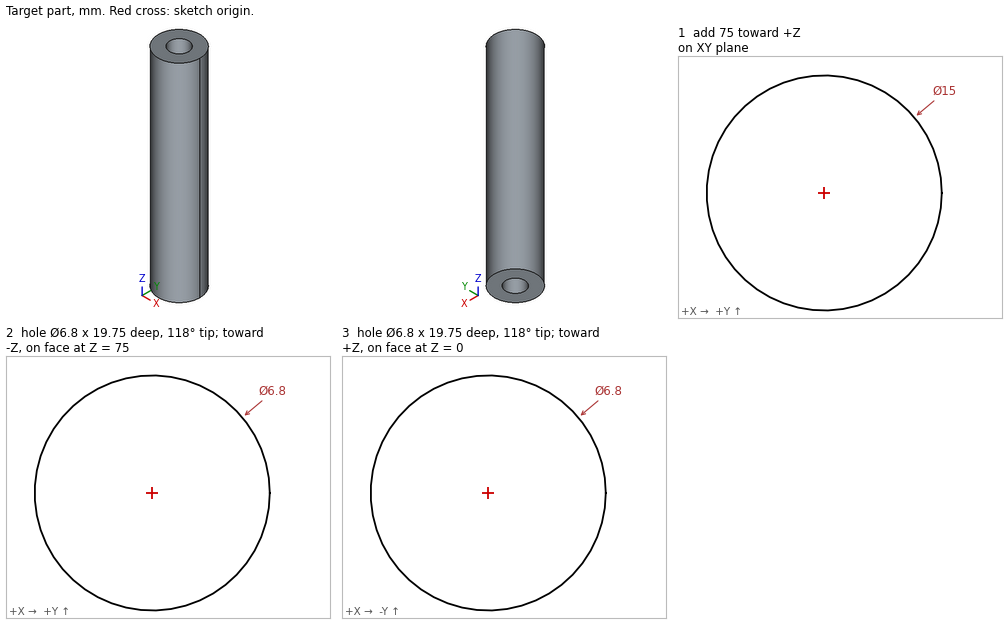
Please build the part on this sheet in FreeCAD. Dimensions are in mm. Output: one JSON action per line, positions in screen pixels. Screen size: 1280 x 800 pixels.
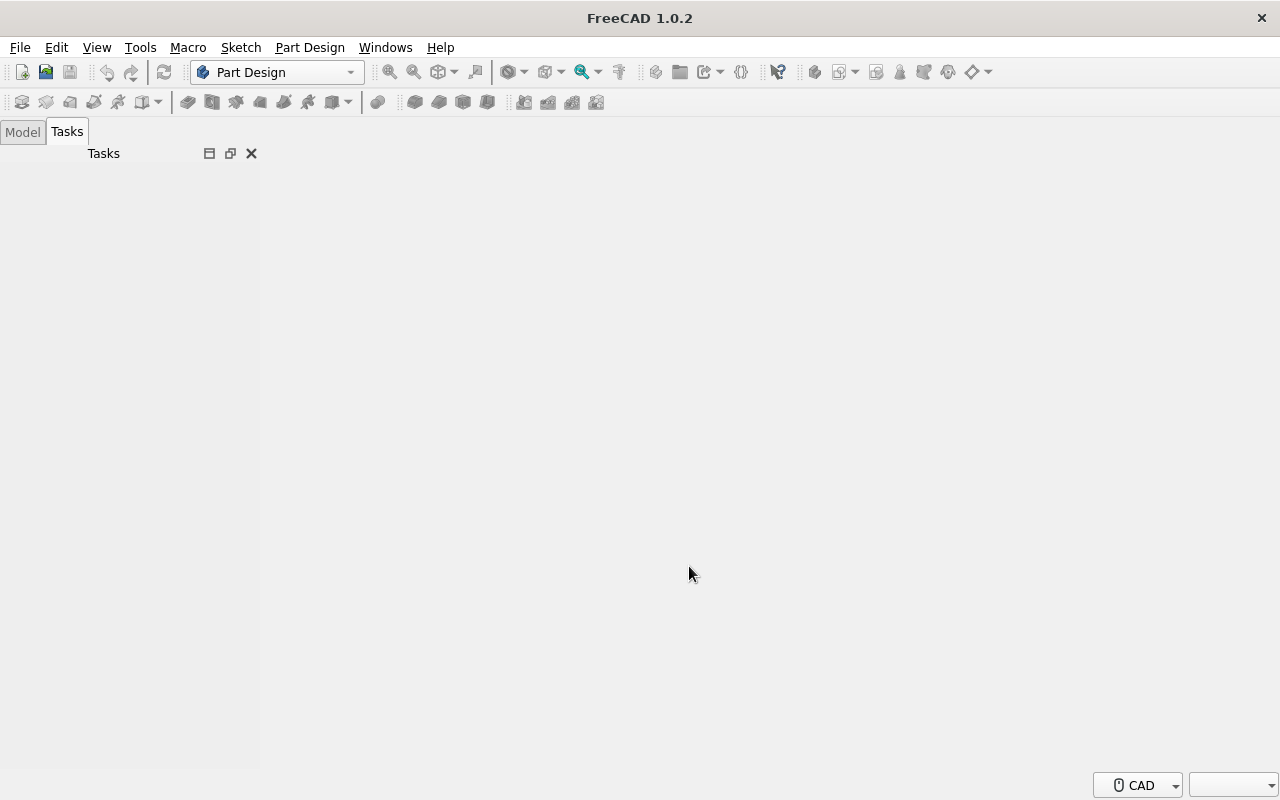
{"action": "left_click", "coordinate": [22, 72]}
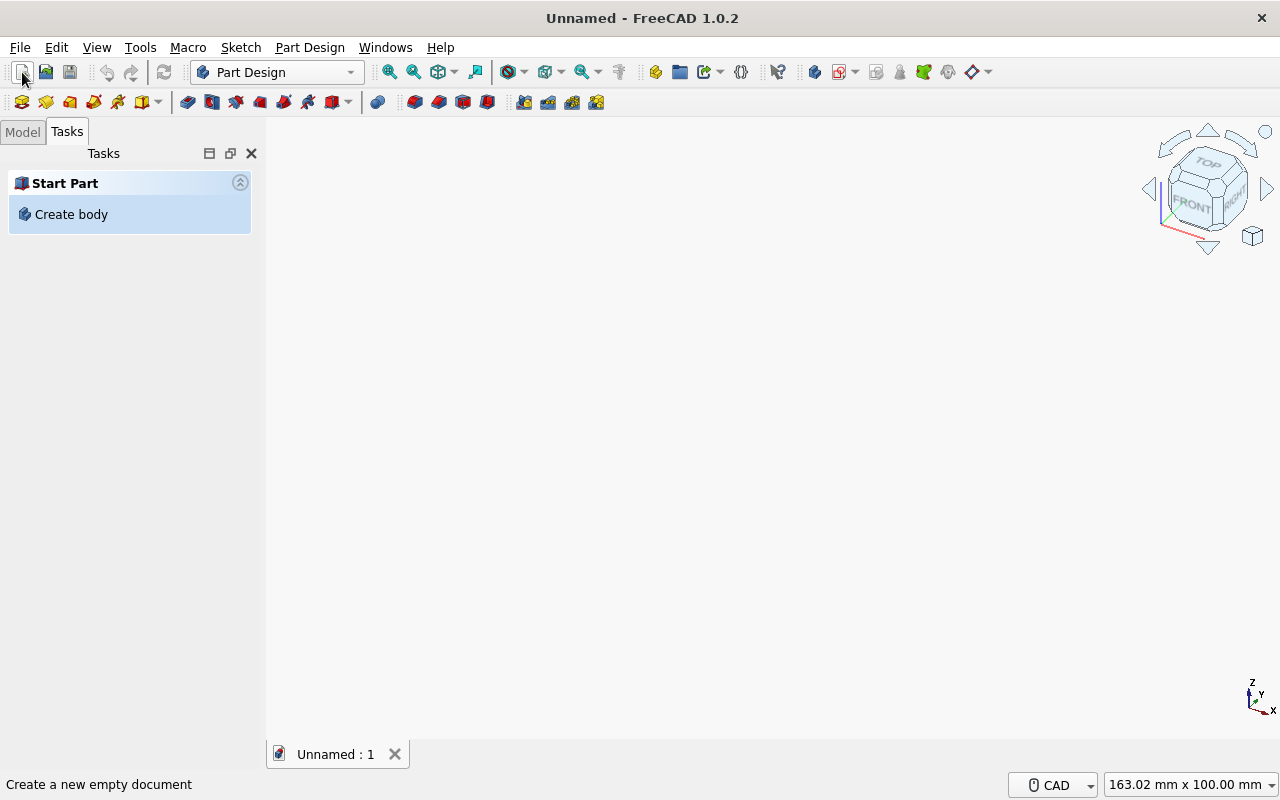
{"action": "left_click", "coordinate": [840, 72]}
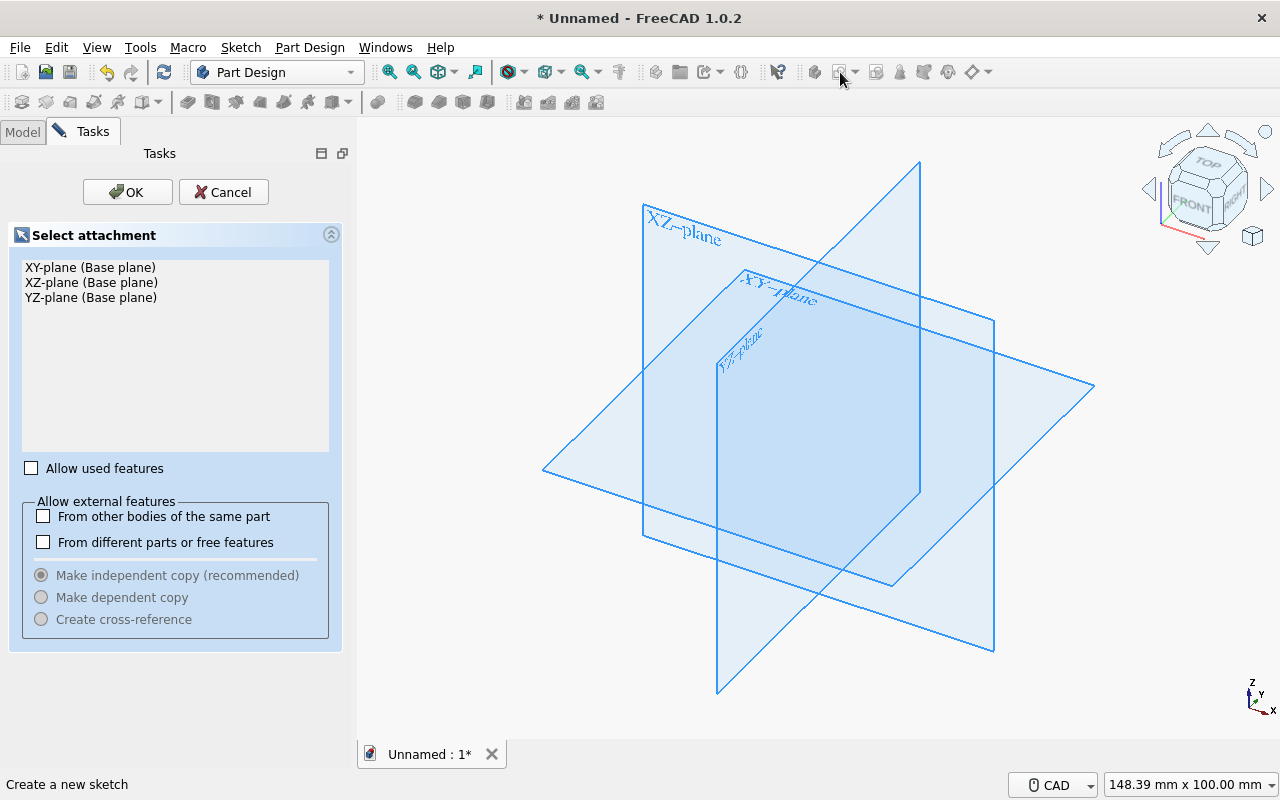
{"action": "left_click", "coordinate": [82, 268]}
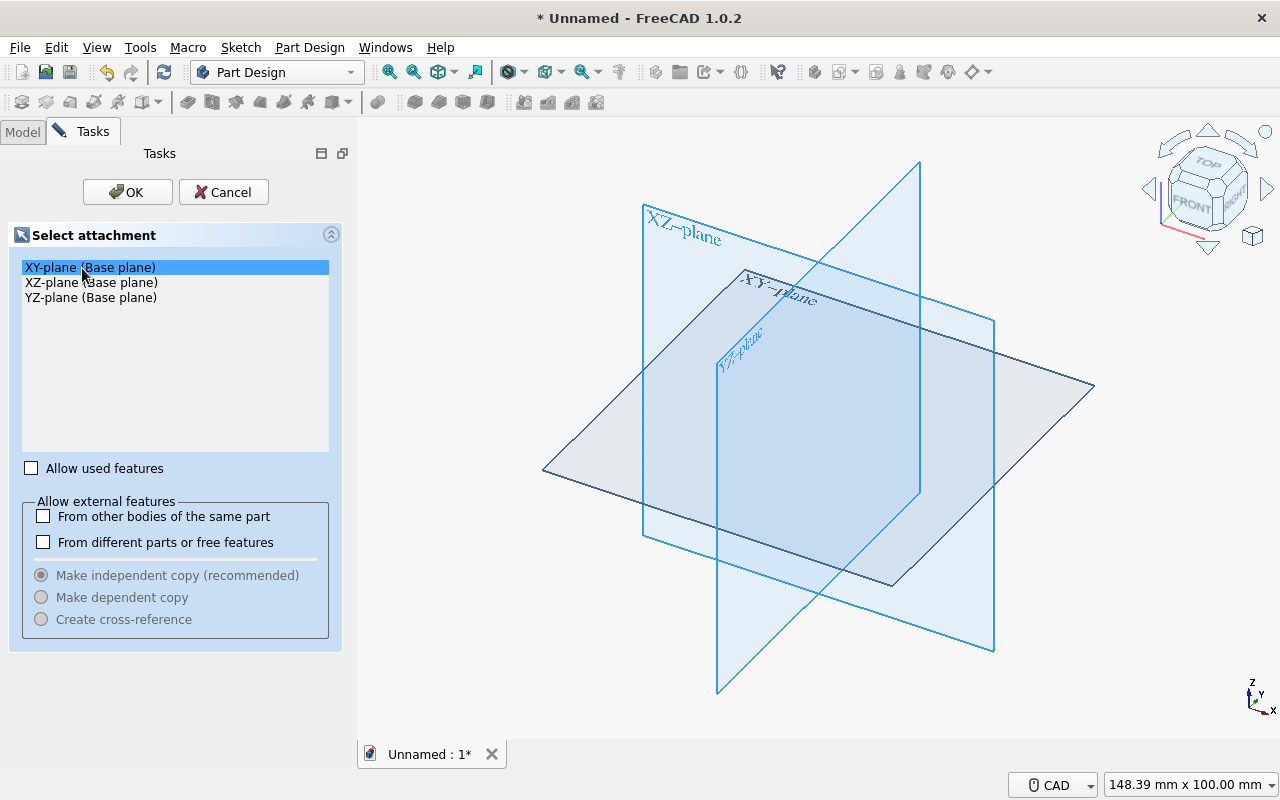
{"action": "left_click", "coordinate": [128, 192]}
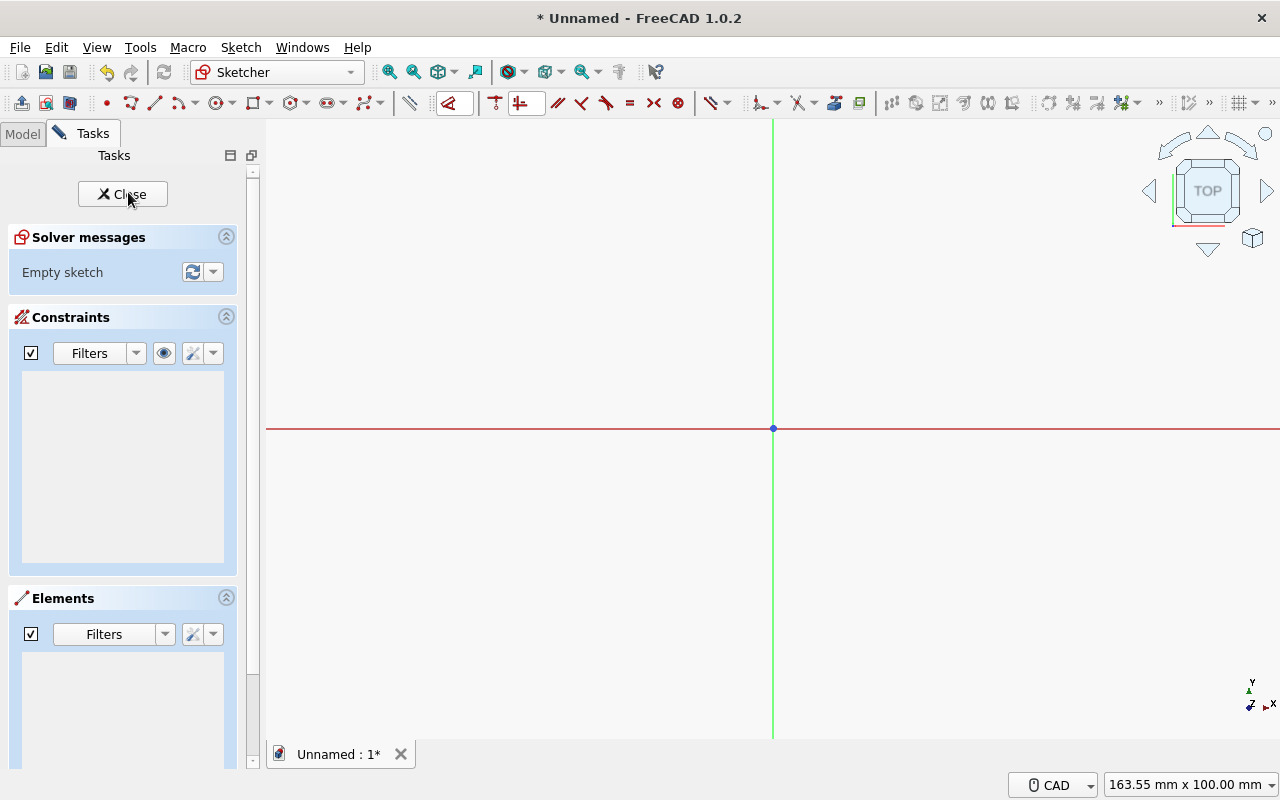
{"action": "scroll", "coordinate": [795, 429], "scroll_direction": "up", "scroll_amount": 7}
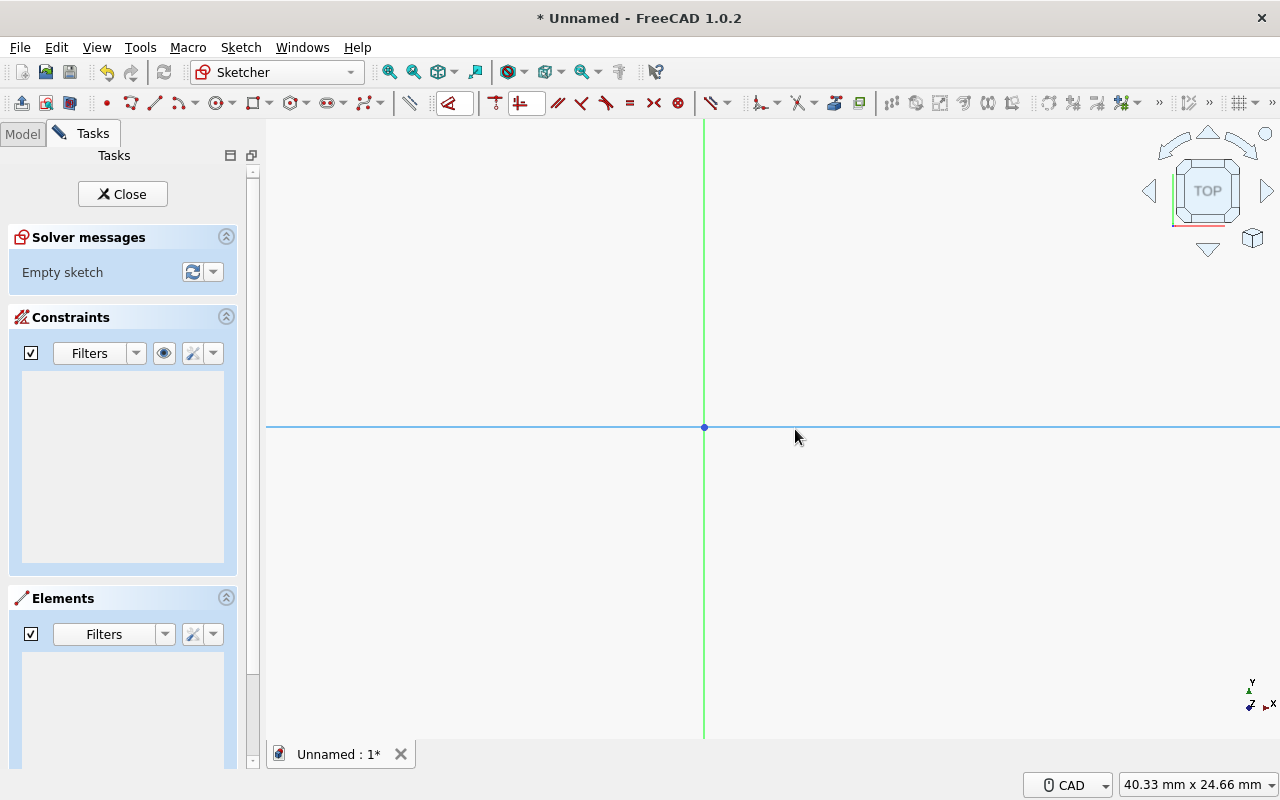
{"action": "left_click", "coordinate": [216, 104]}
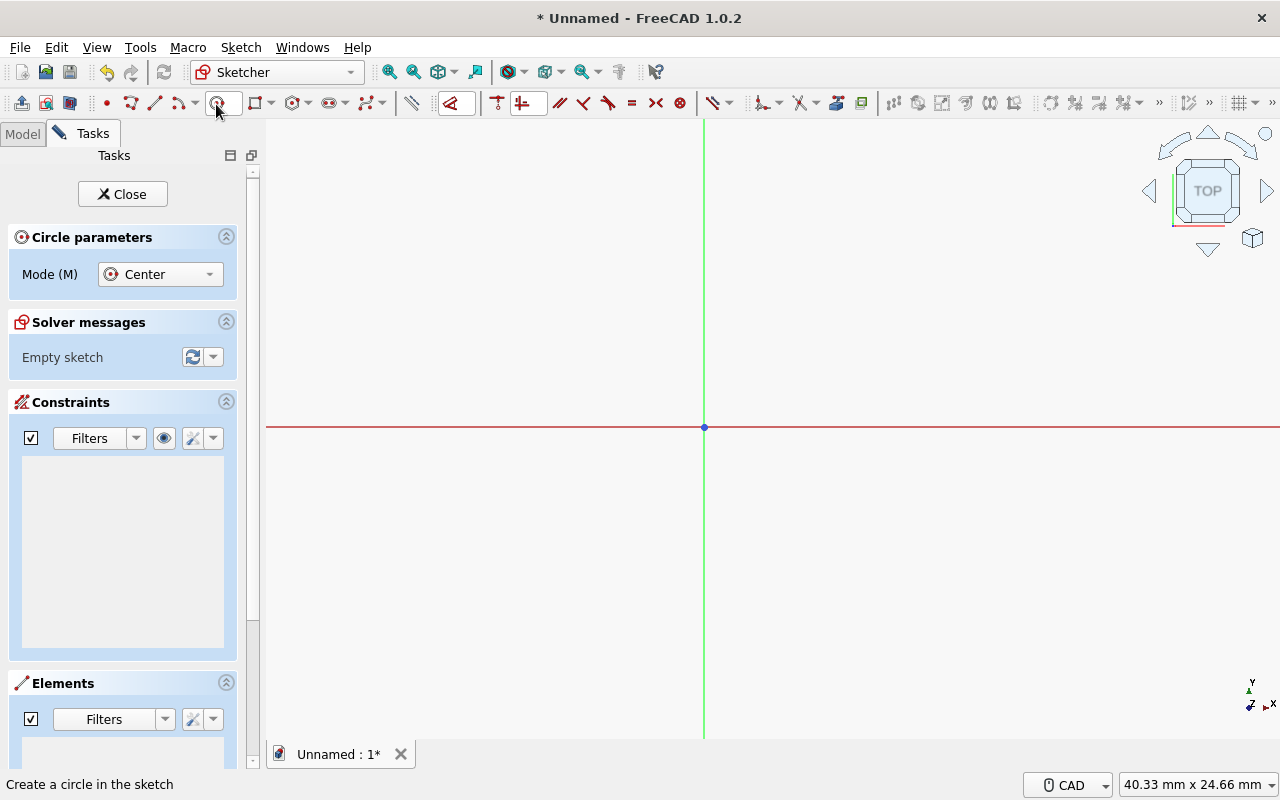
{"action": "left_click", "coordinate": [704, 427]}
{"action": "mouse_move", "coordinate": [838, 294]}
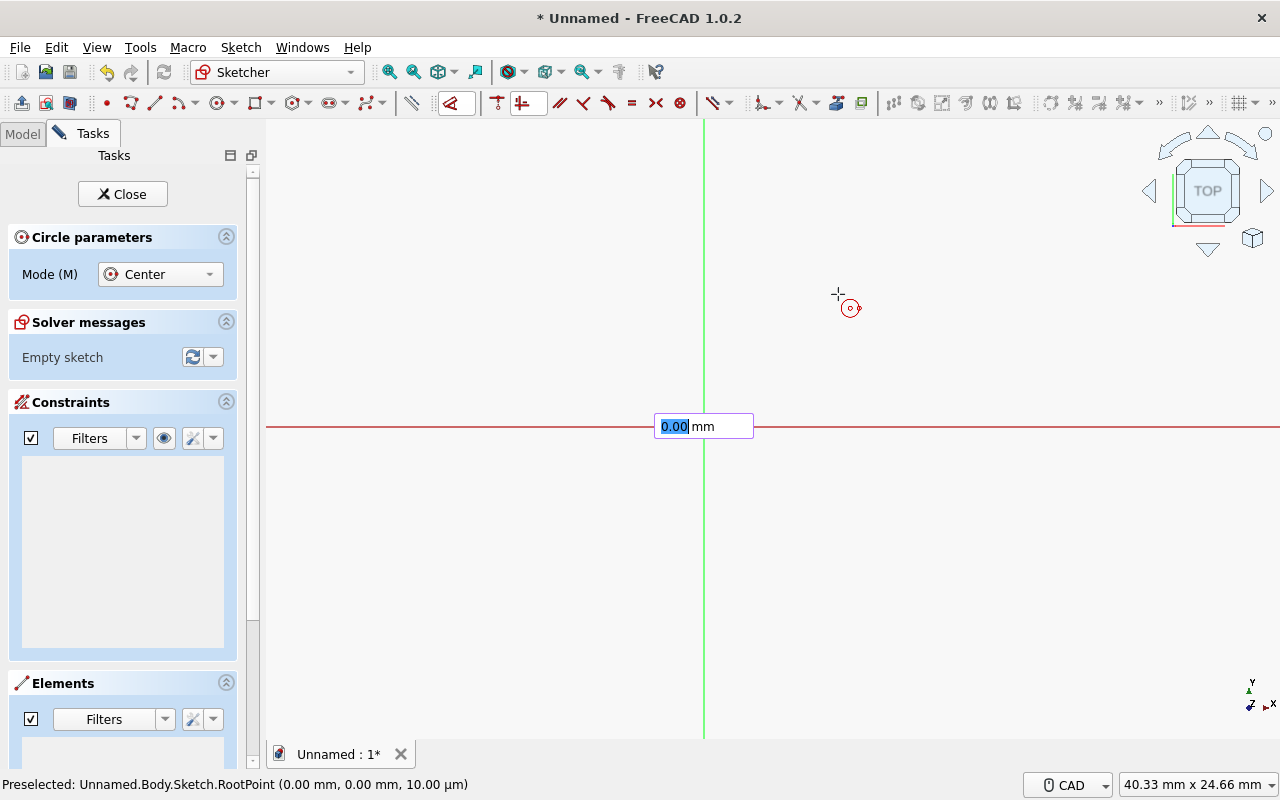
{"action": "type", "text": "15"}
{"action": "key", "text": "Return"}
{"action": "key", "text": "Escape"}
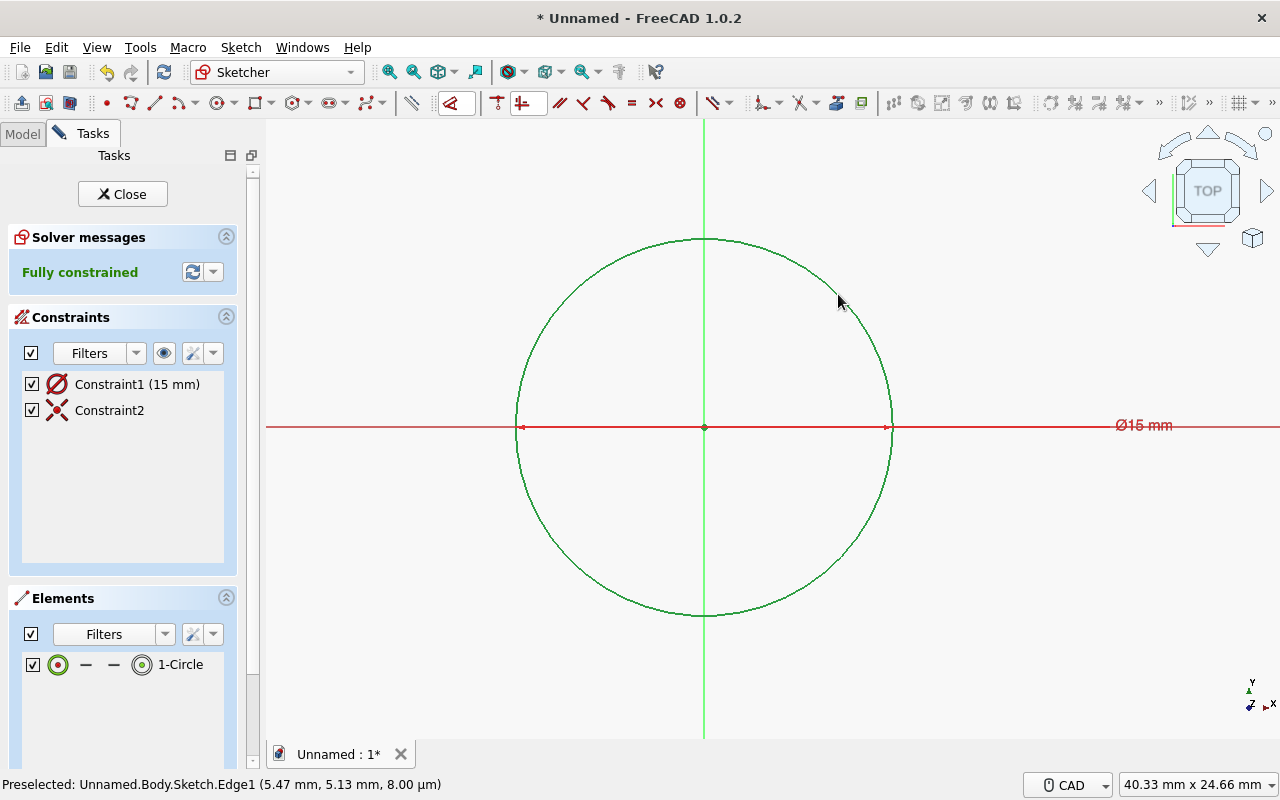
{"action": "left_click", "coordinate": [123, 194]}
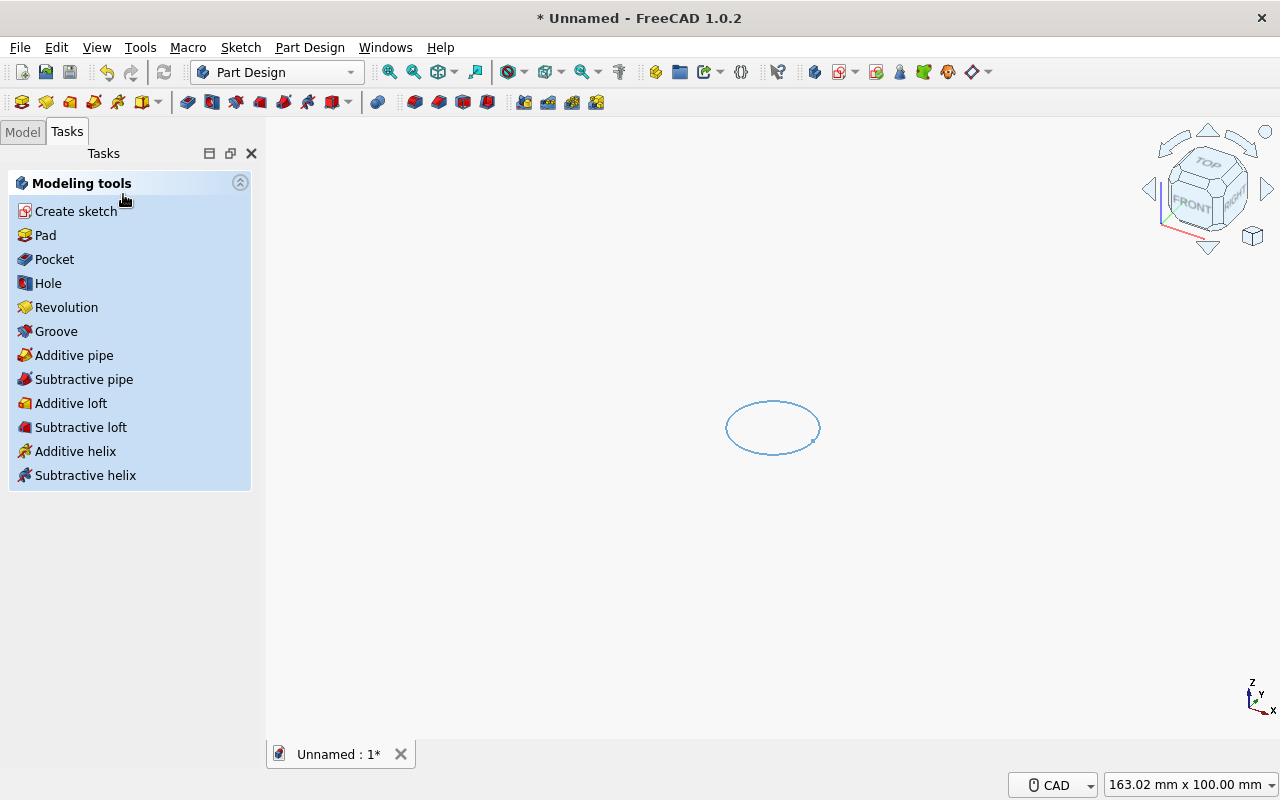
{"action": "left_click", "coordinate": [22, 102]}